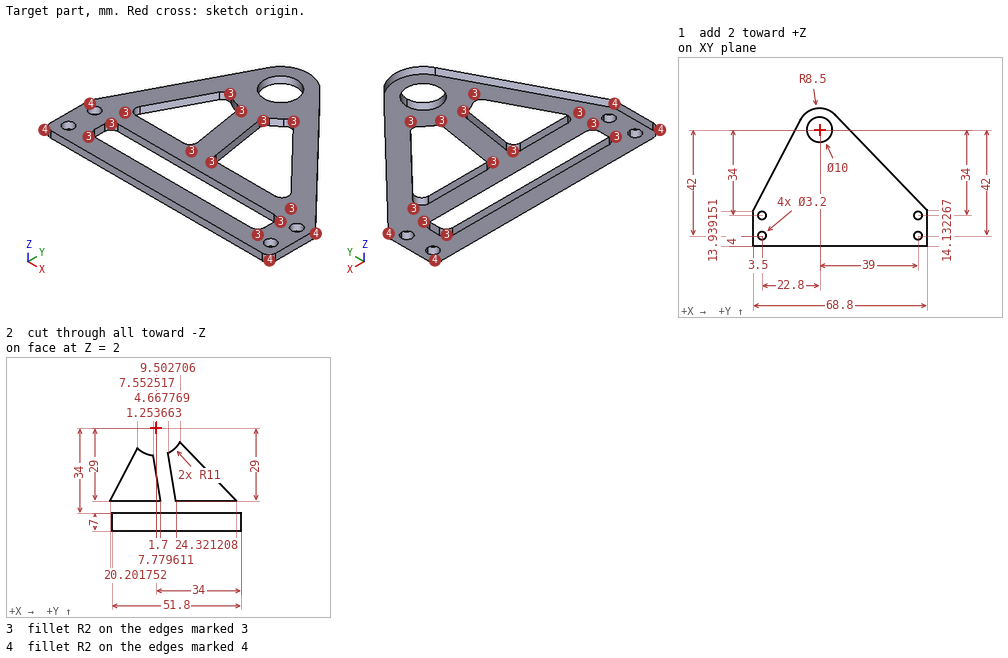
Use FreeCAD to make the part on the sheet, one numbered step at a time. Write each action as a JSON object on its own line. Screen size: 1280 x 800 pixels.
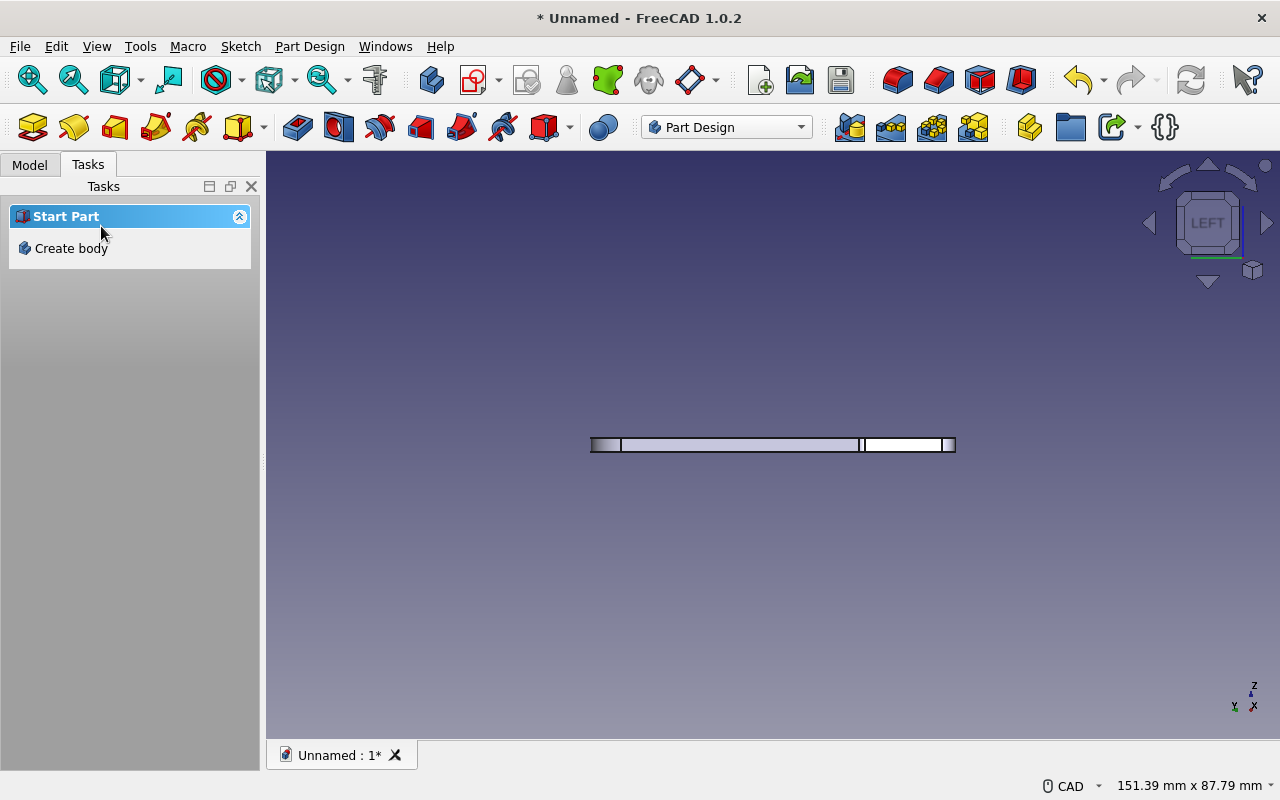
{"action": "key", "text": "0"}